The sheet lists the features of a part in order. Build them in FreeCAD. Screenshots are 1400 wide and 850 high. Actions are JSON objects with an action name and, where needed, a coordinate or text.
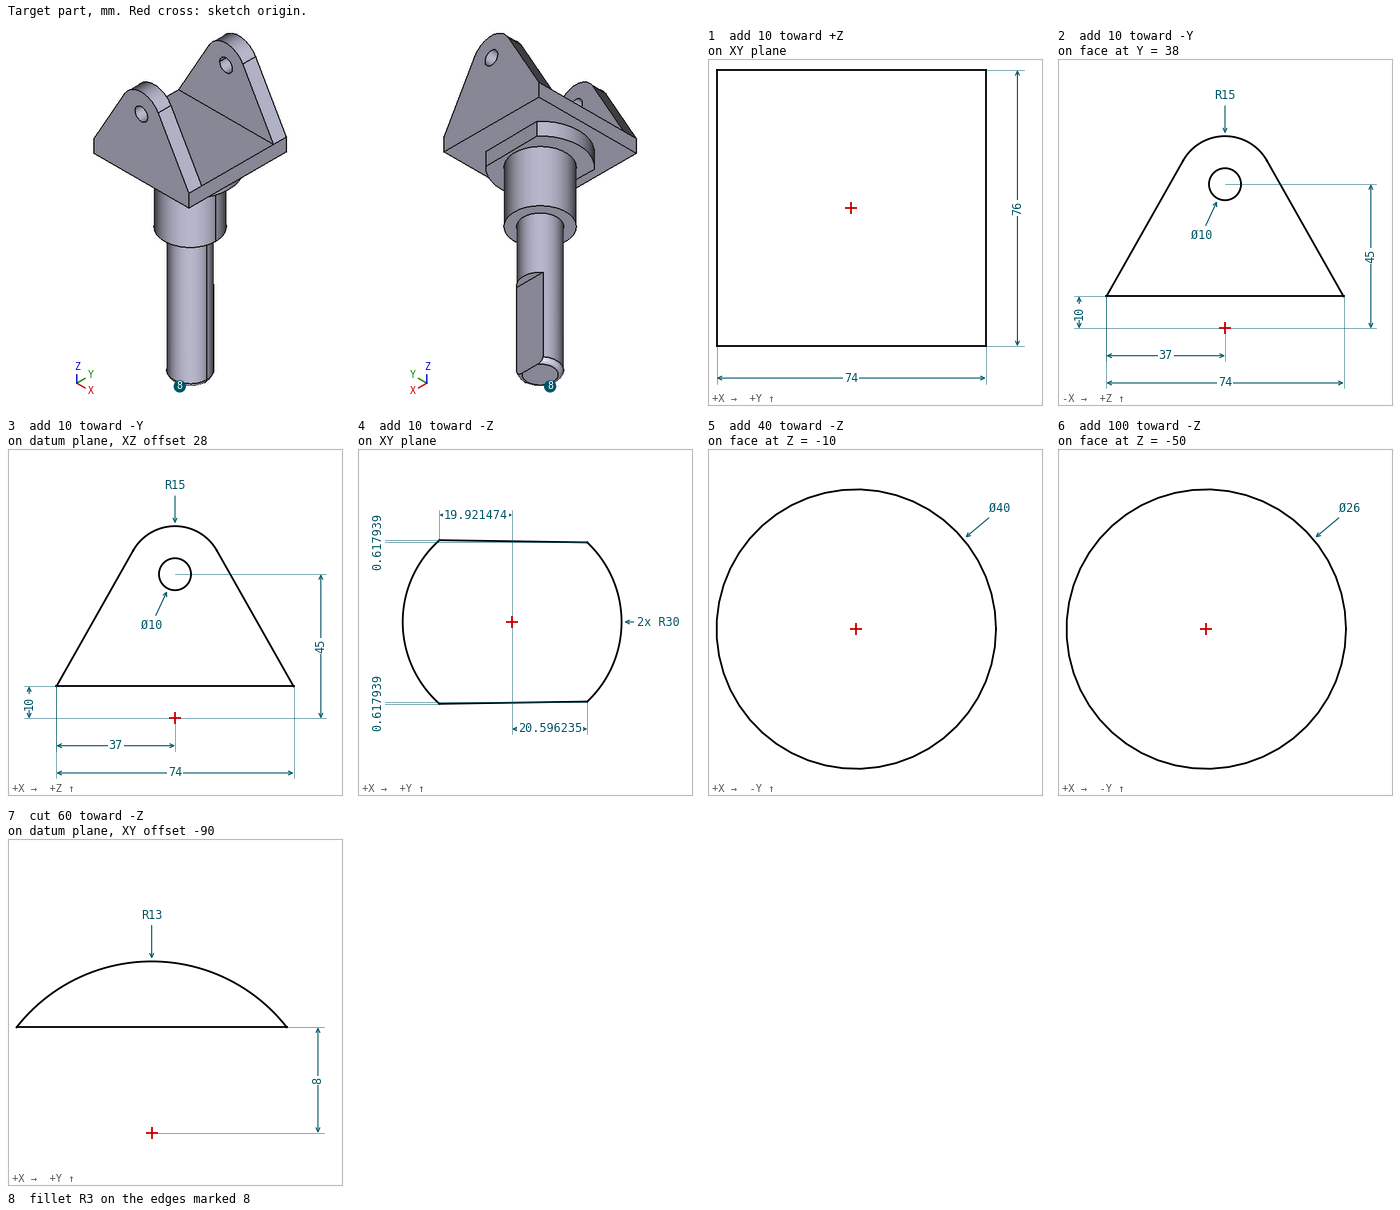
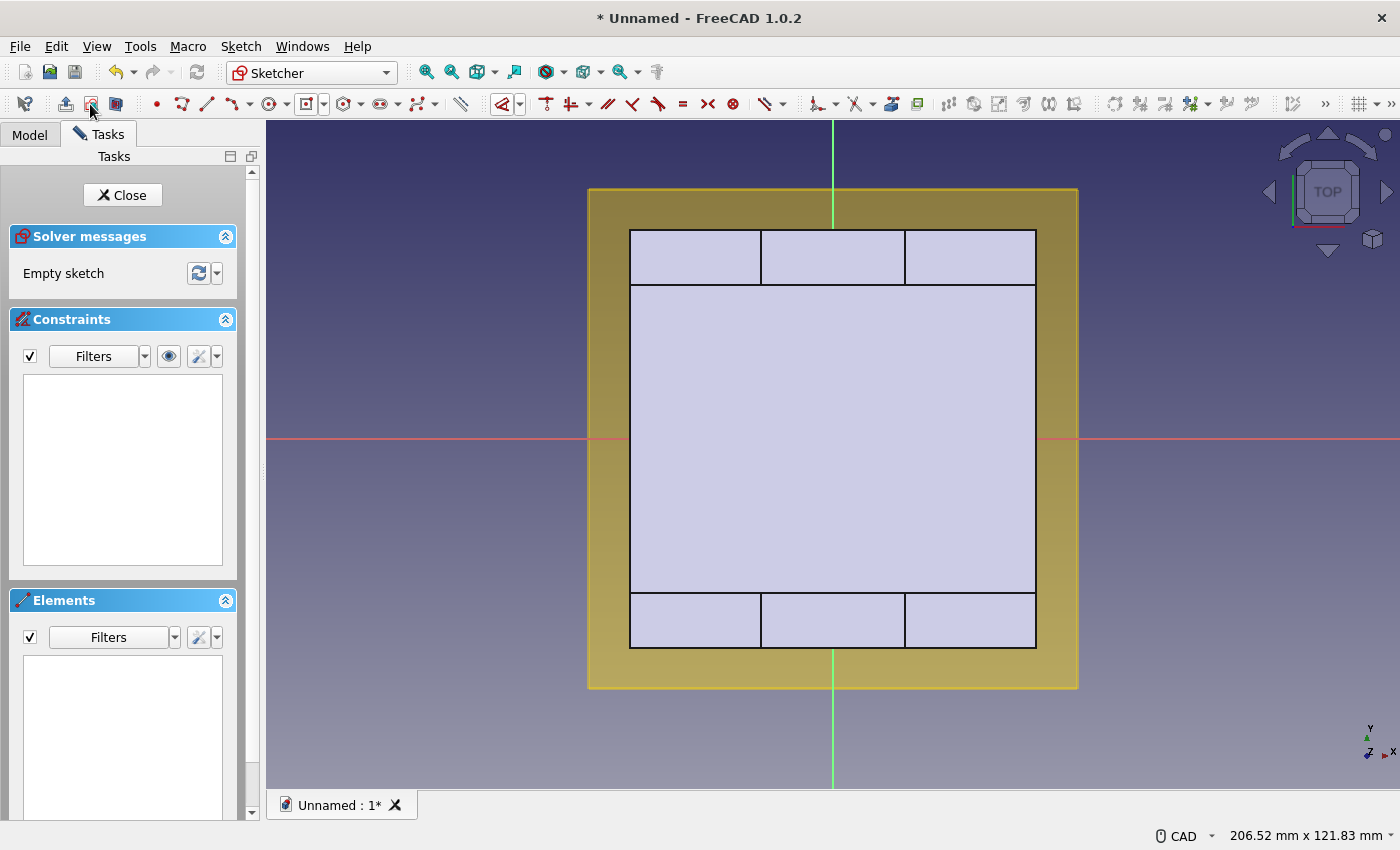
{"action": "left_click", "coordinate": [116, 104]}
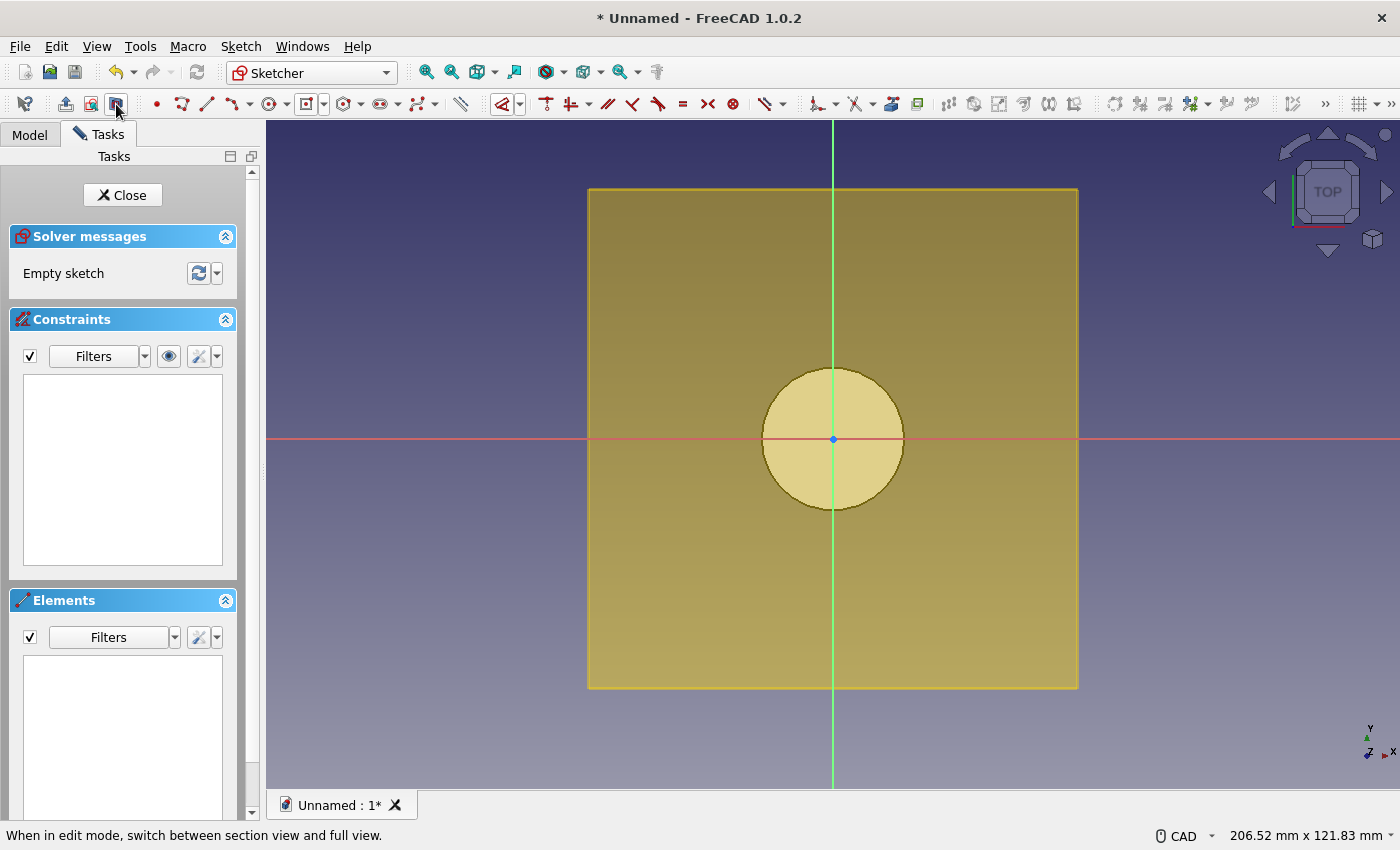
{"action": "scroll", "coordinate": [847, 393], "scroll_direction": "up", "scroll_amount": 9}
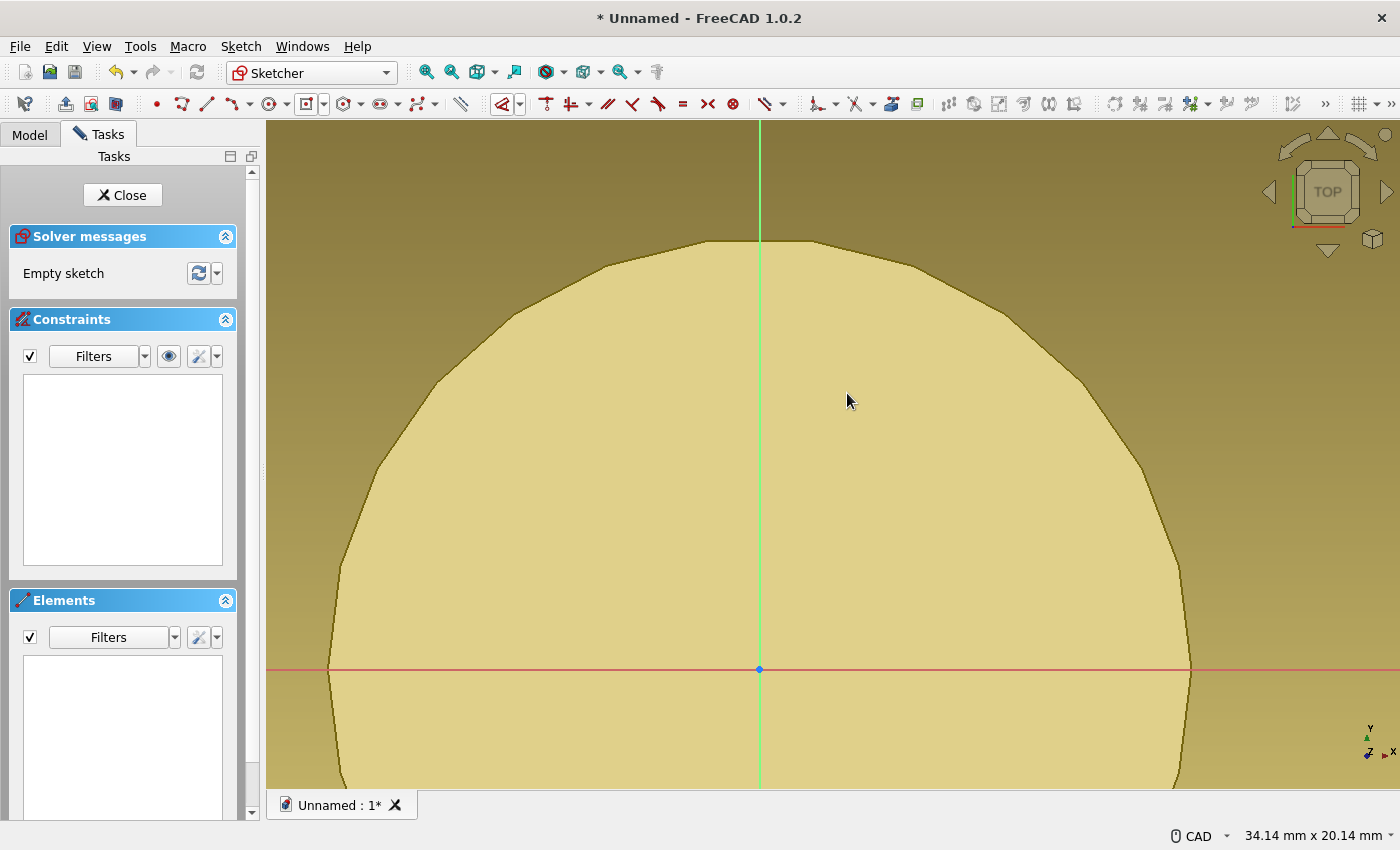
{"action": "left_click", "coordinate": [207, 104]}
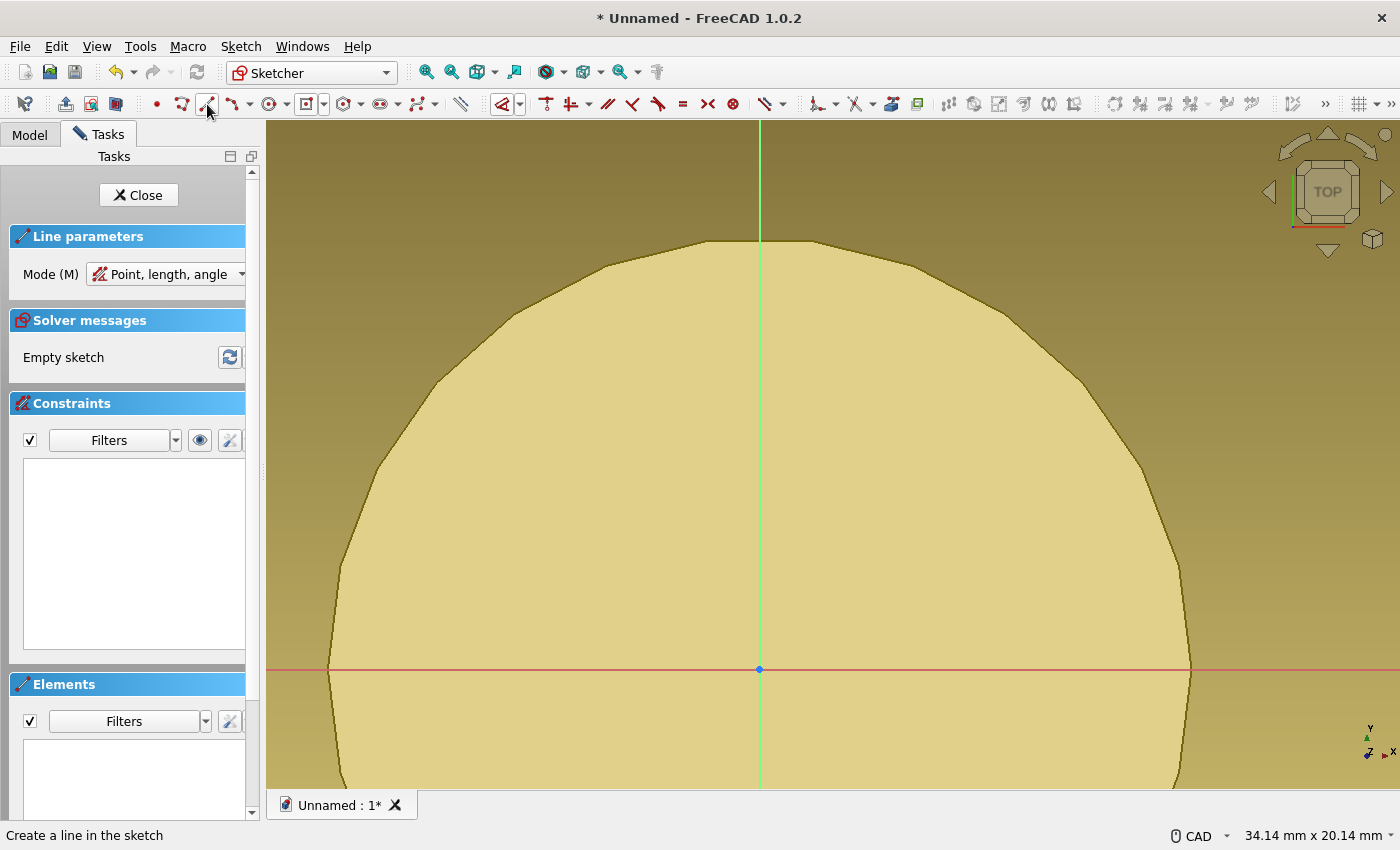
{"action": "left_click", "coordinate": [1100, 404]}
{"action": "left_click", "coordinate": [419, 404]}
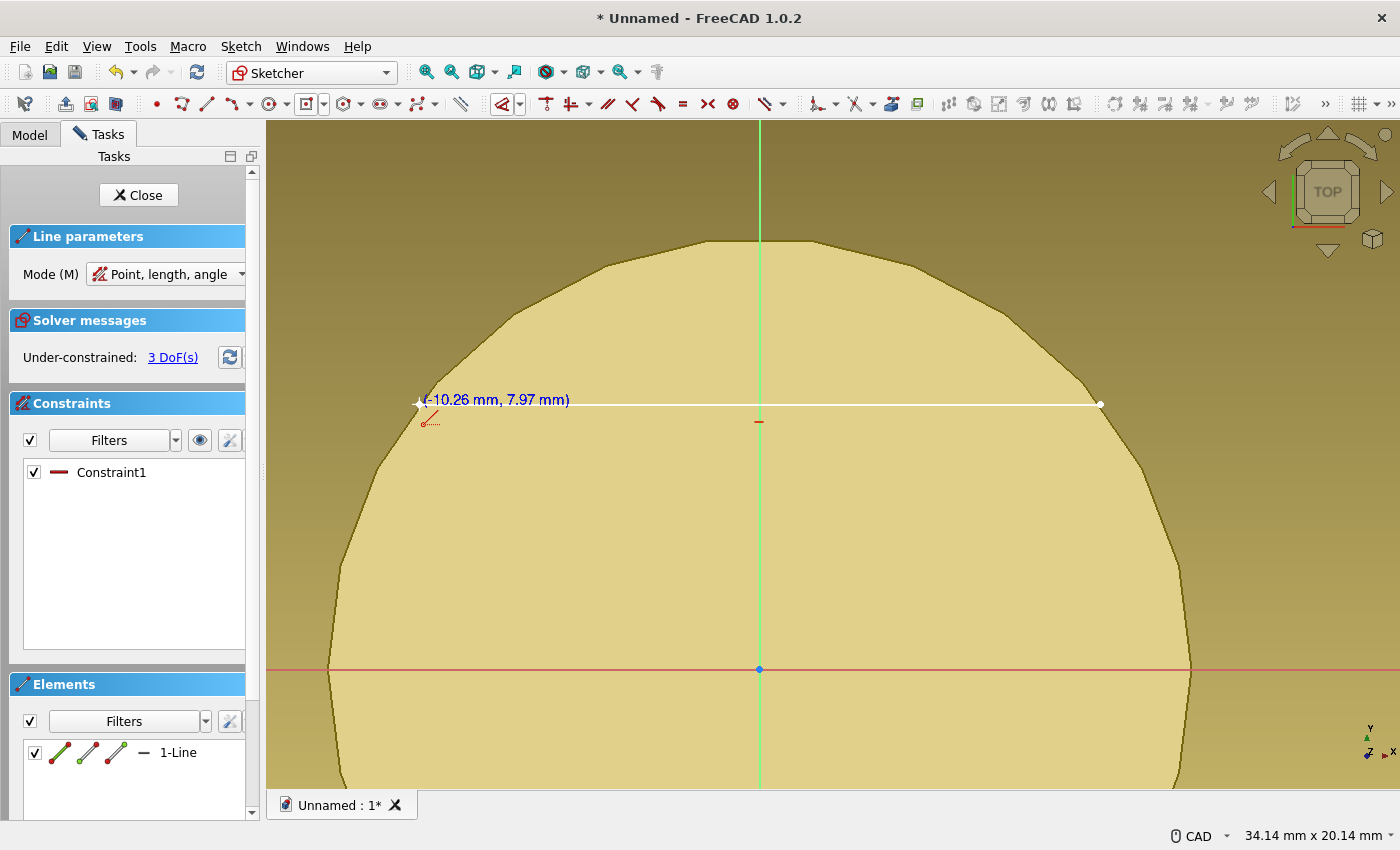
{"action": "left_click", "coordinate": [232, 104]}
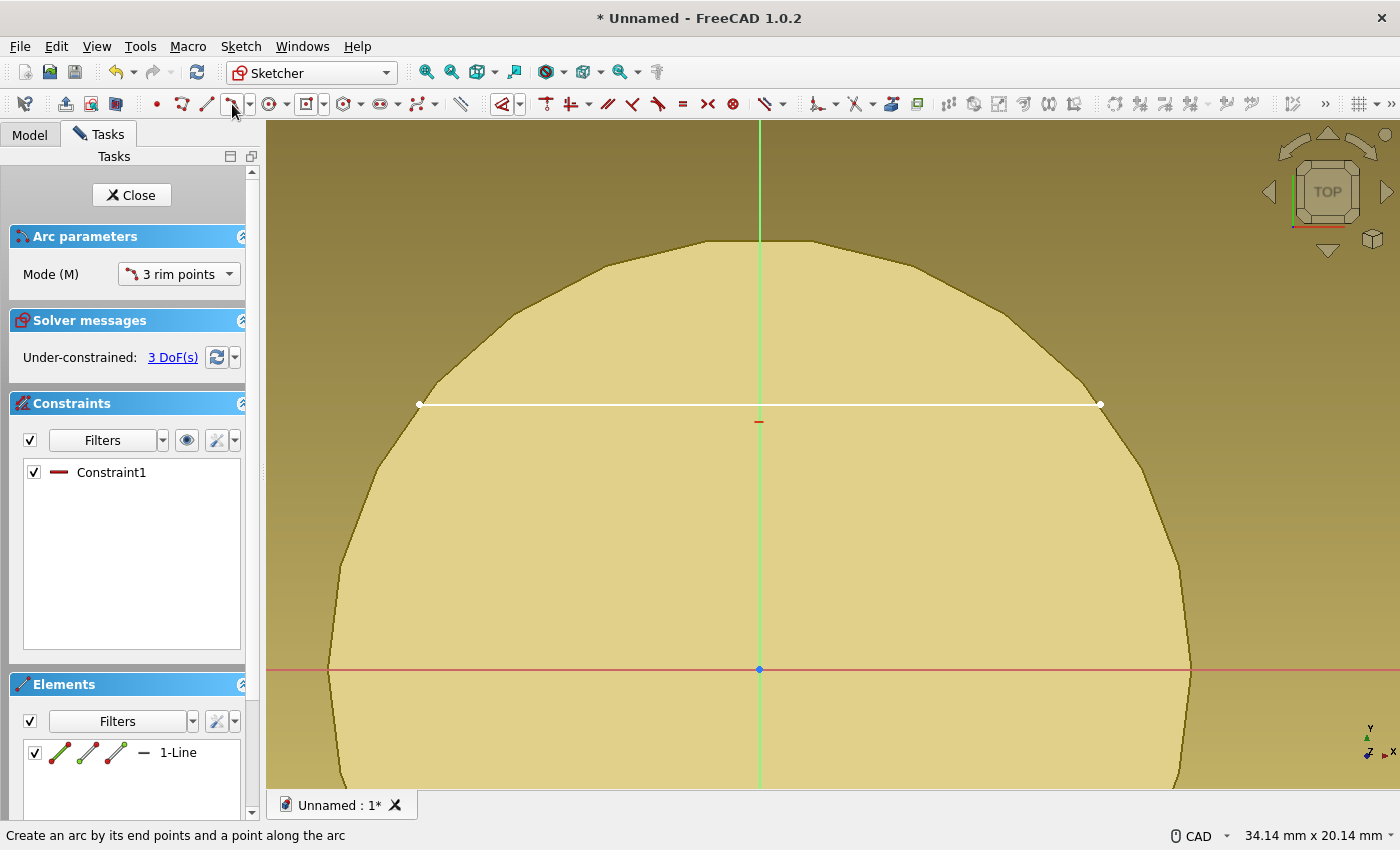
{"action": "left_click", "coordinate": [419, 405]}
{"action": "left_click", "coordinate": [1100, 405]}
{"action": "left_click", "coordinate": [838, 245]}
{"action": "key", "text": "Escape"}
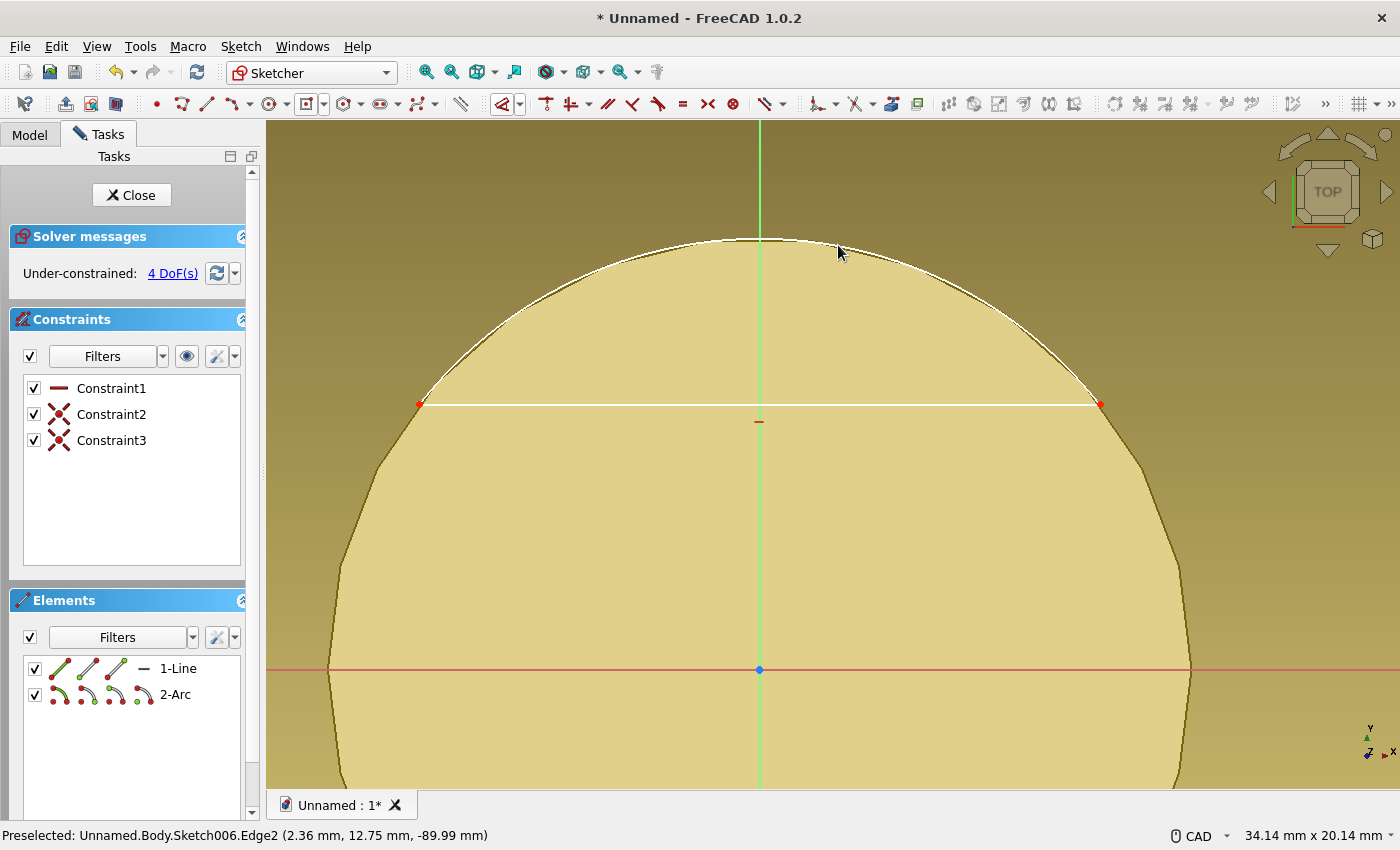
{"action": "left_click_drag", "start_coordinate": [750, 660], "coordinate": [770, 681]}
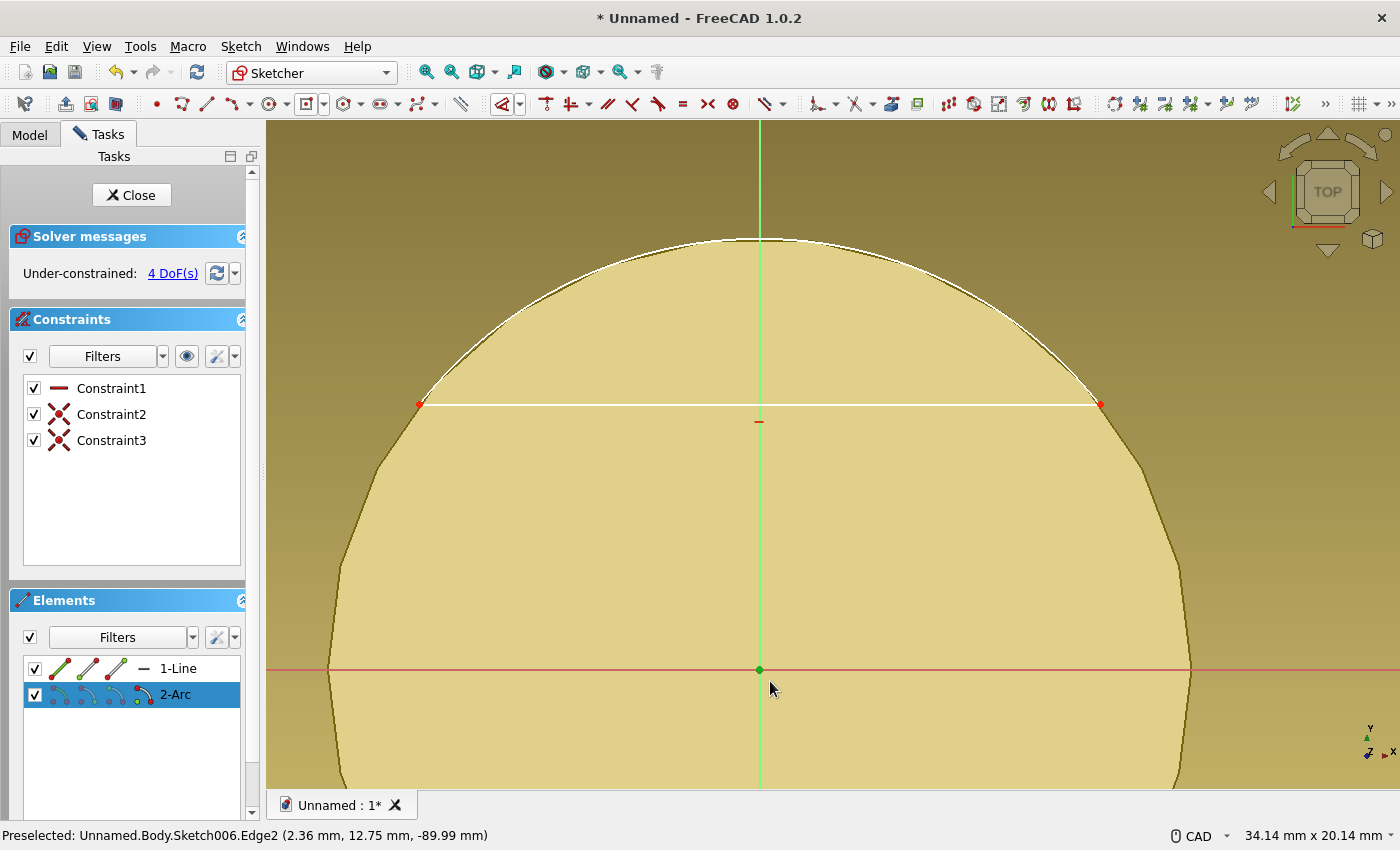
{"action": "left_click", "coordinate": [546, 104]}